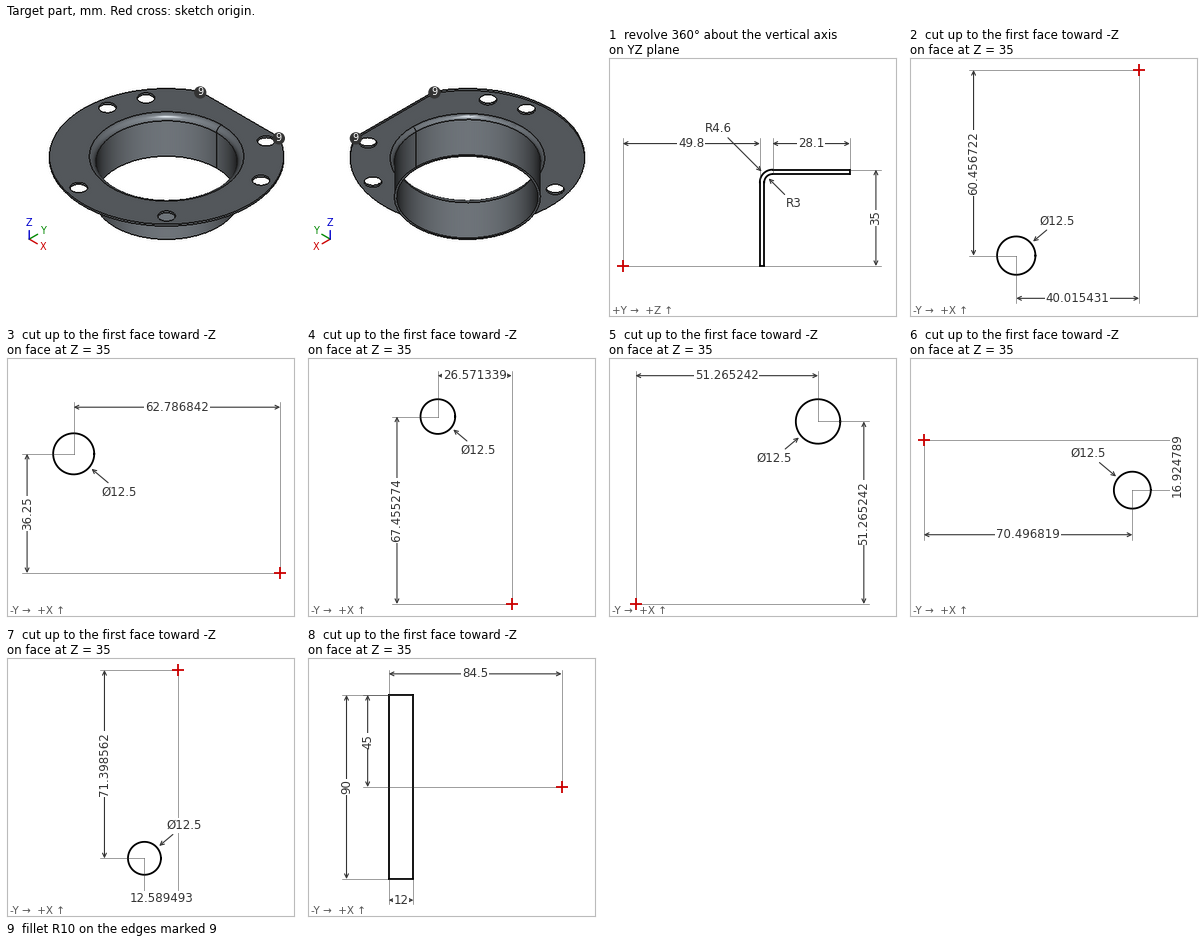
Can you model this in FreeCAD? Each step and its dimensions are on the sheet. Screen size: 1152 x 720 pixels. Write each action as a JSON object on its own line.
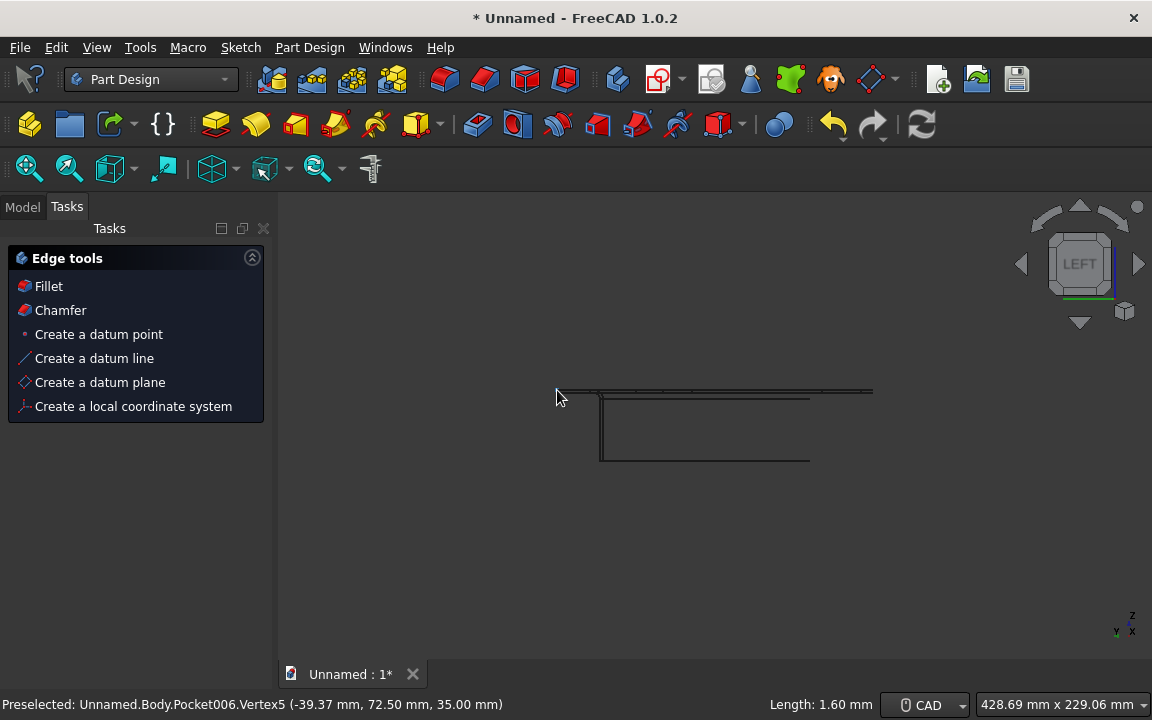
{"action": "key", "text": "0"}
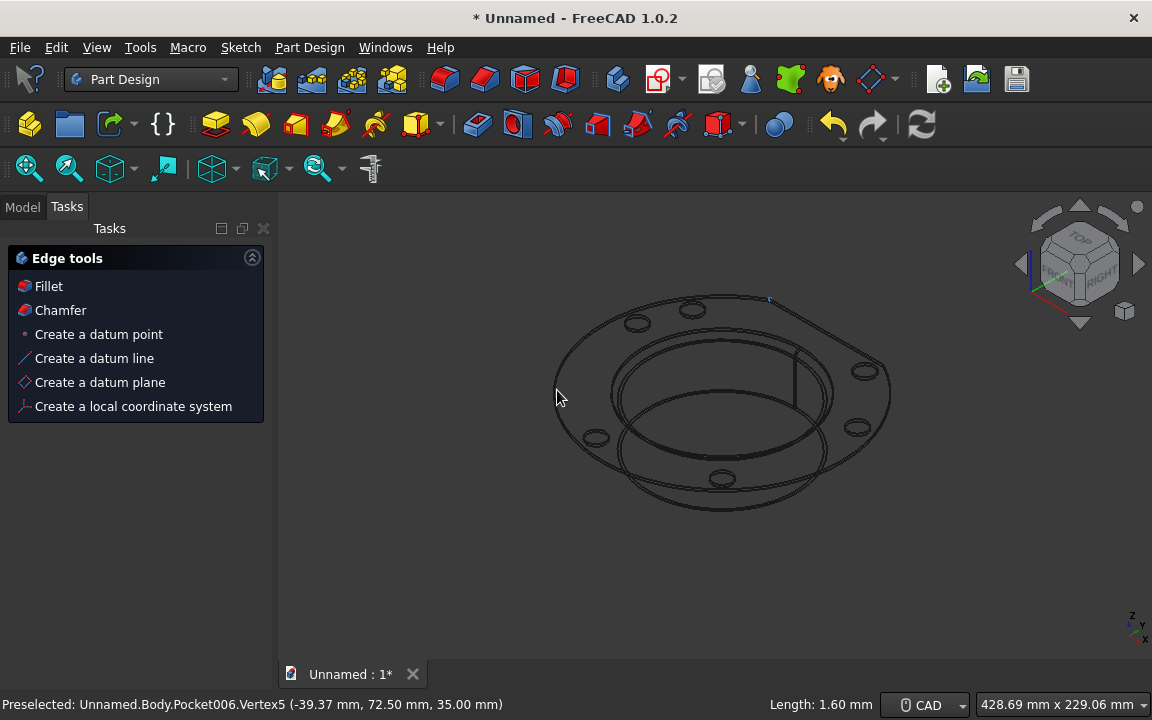
{"action": "scroll", "coordinate": [883, 365], "scroll_direction": "up", "scroll_amount": 13}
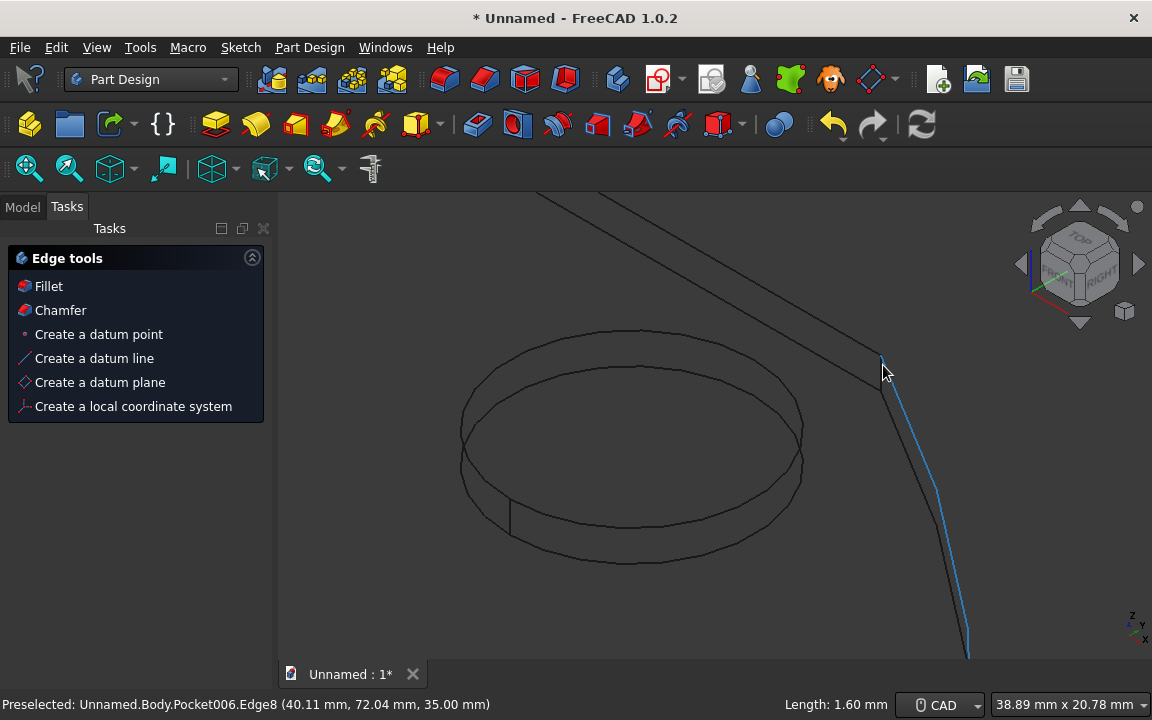
{"action": "left_click", "coordinate": [881, 372], "text": "ctrl"}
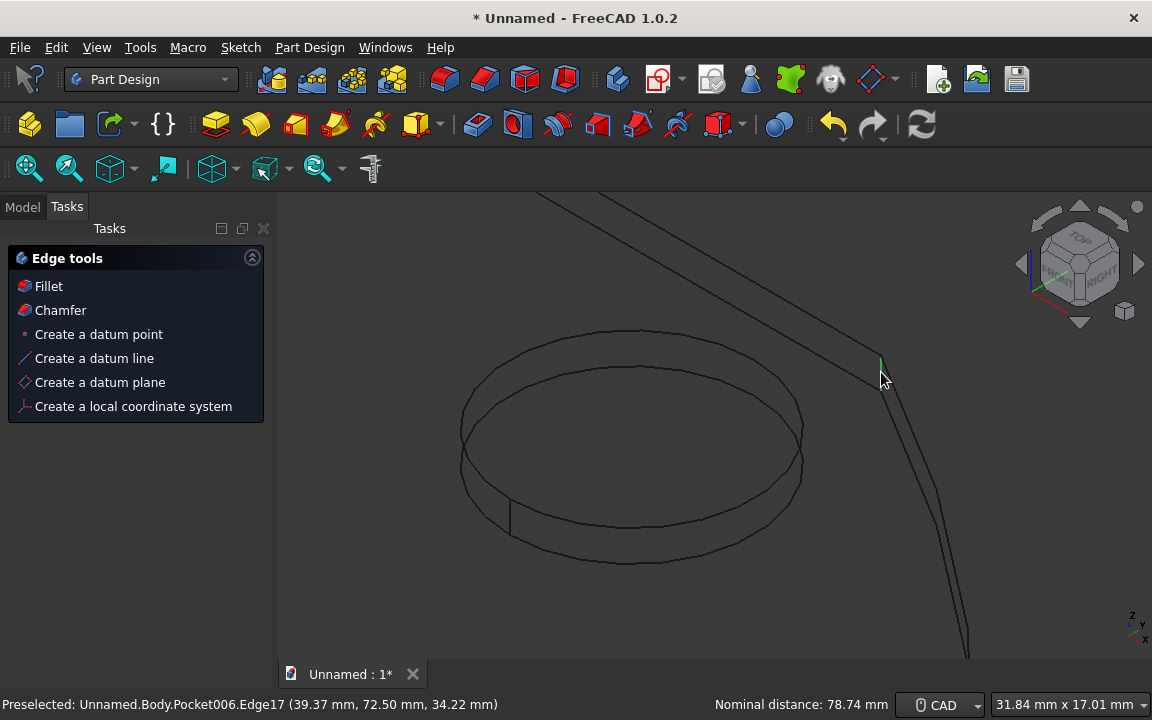
{"action": "key", "text": "v 1"}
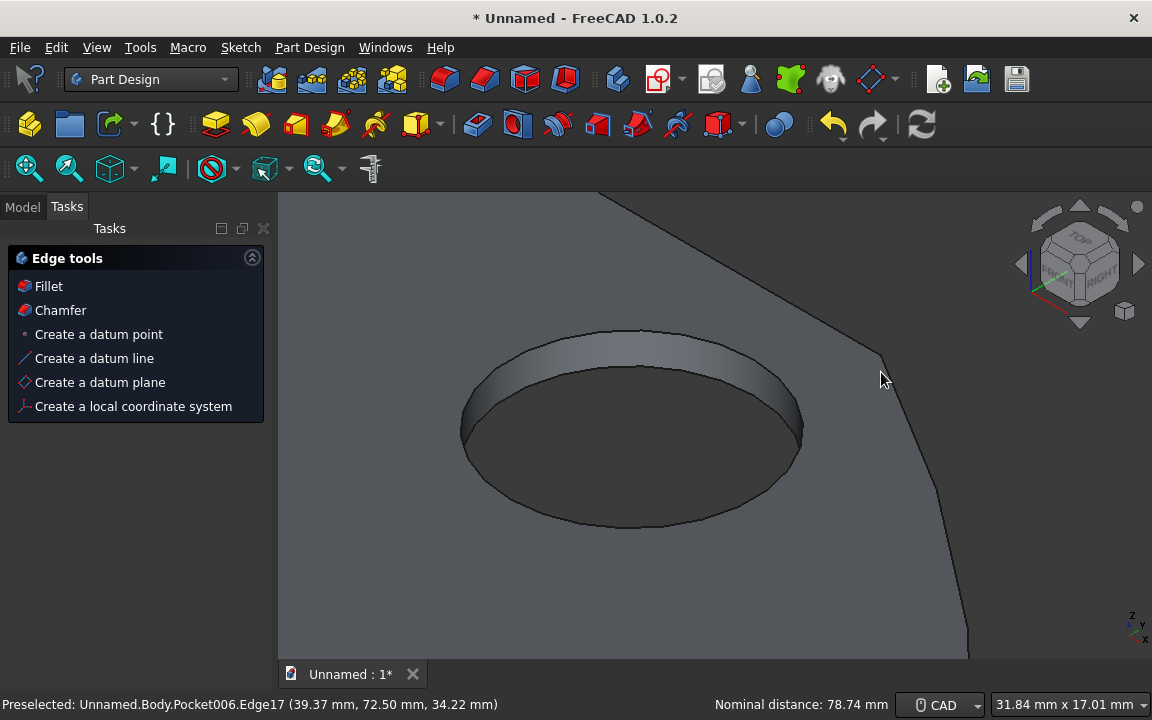
{"action": "left_click", "coordinate": [446, 80]}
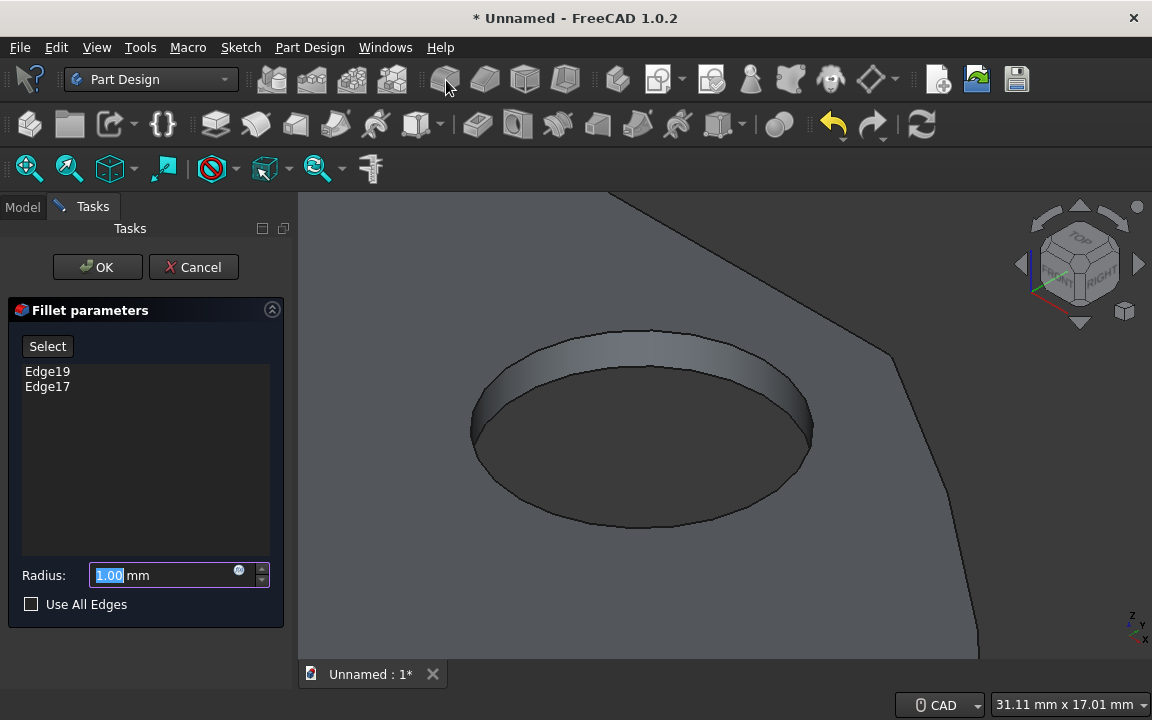
{"action": "type", "text": "10"}
{"action": "key", "text": "Tab"}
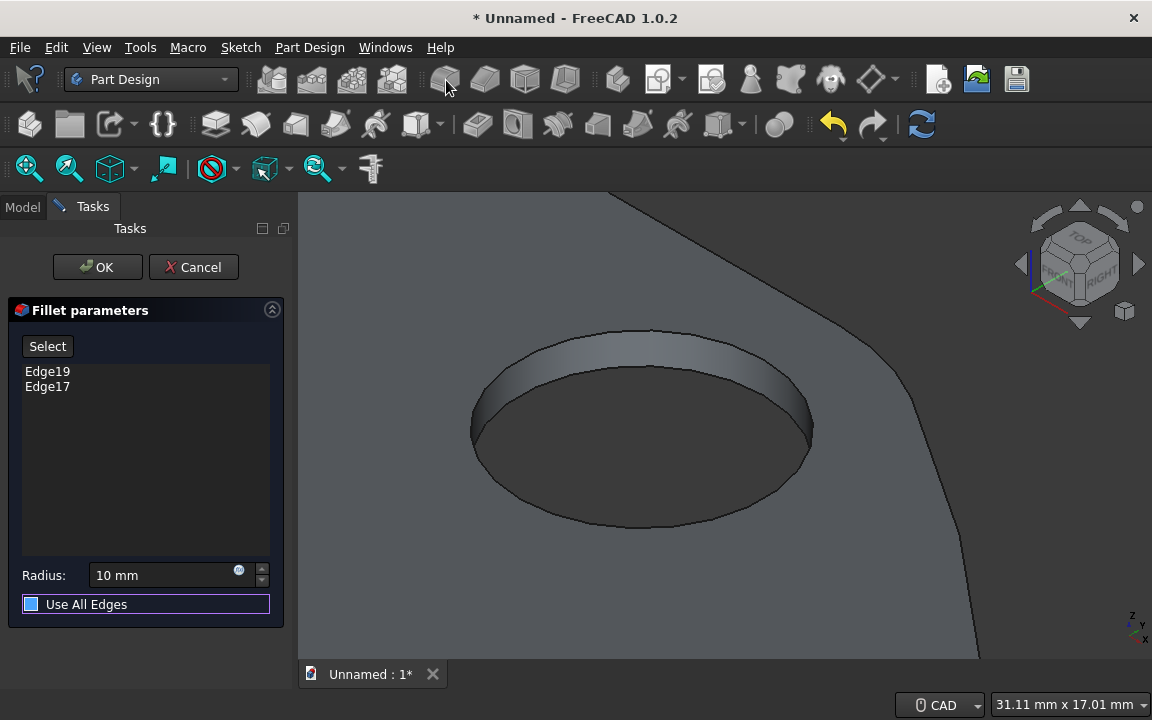
{"action": "left_click", "coordinate": [98, 267]}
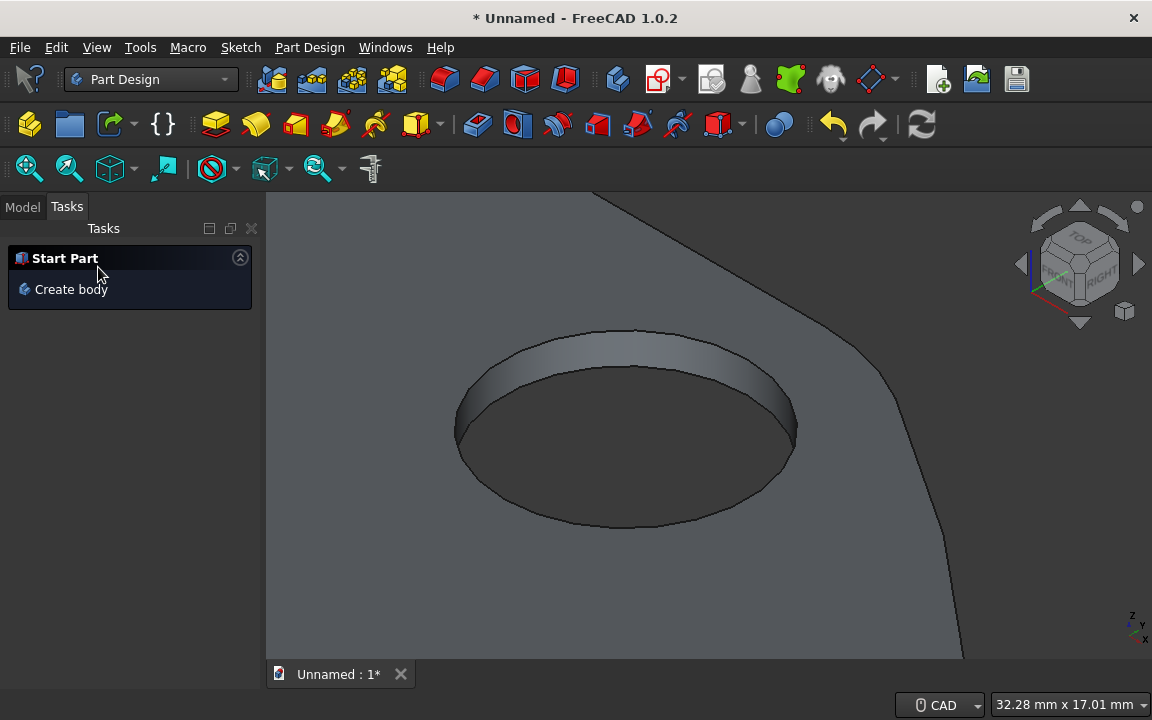
{"action": "left_click", "coordinate": [30, 170]}